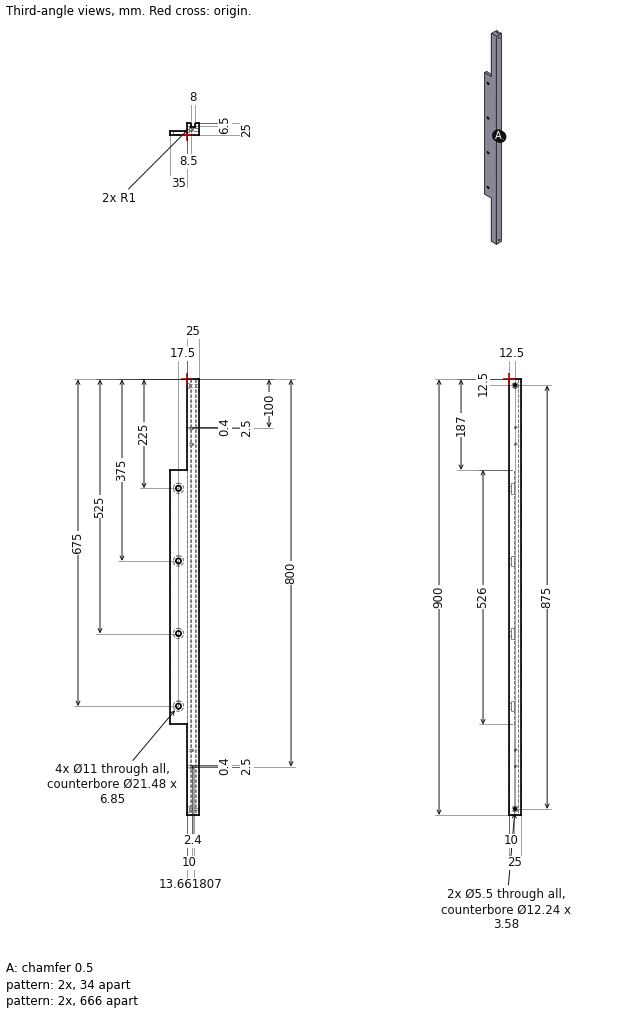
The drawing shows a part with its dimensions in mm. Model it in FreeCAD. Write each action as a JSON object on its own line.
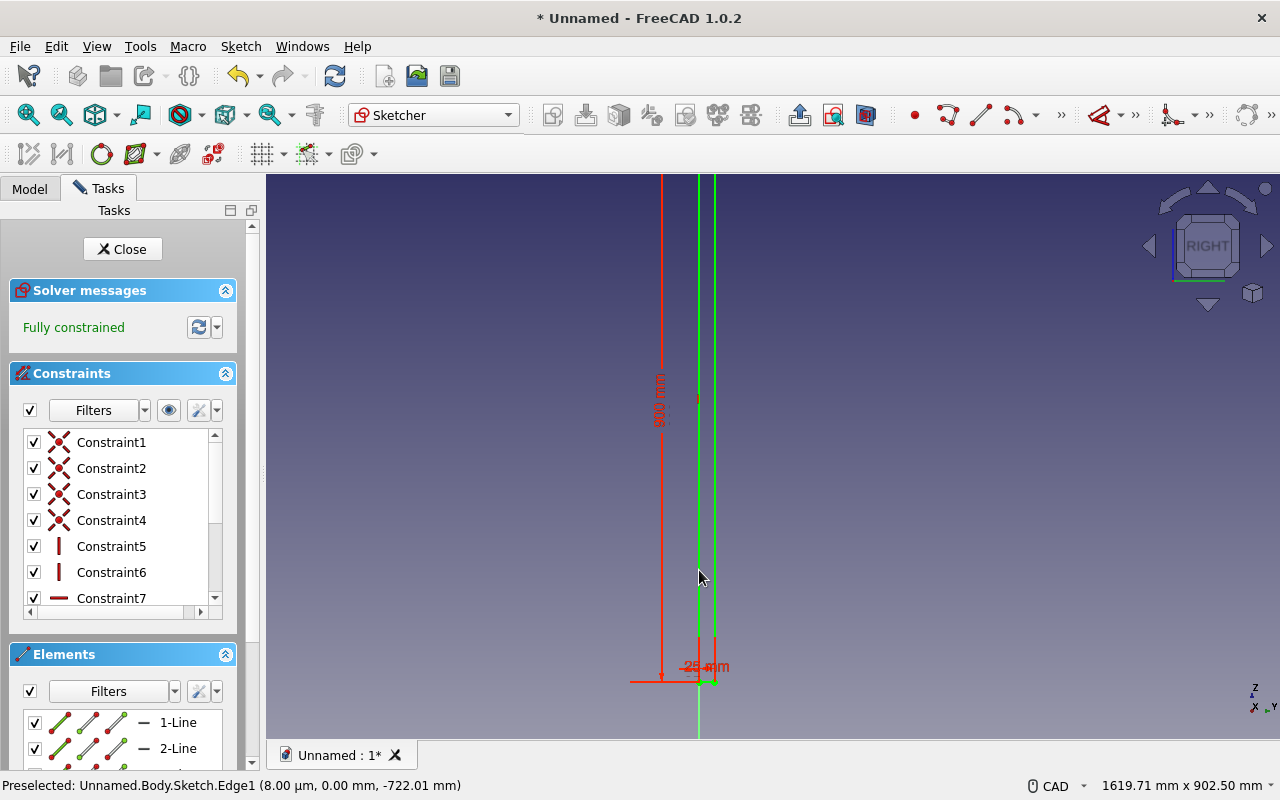
{"action": "left_click", "coordinate": [123, 249]}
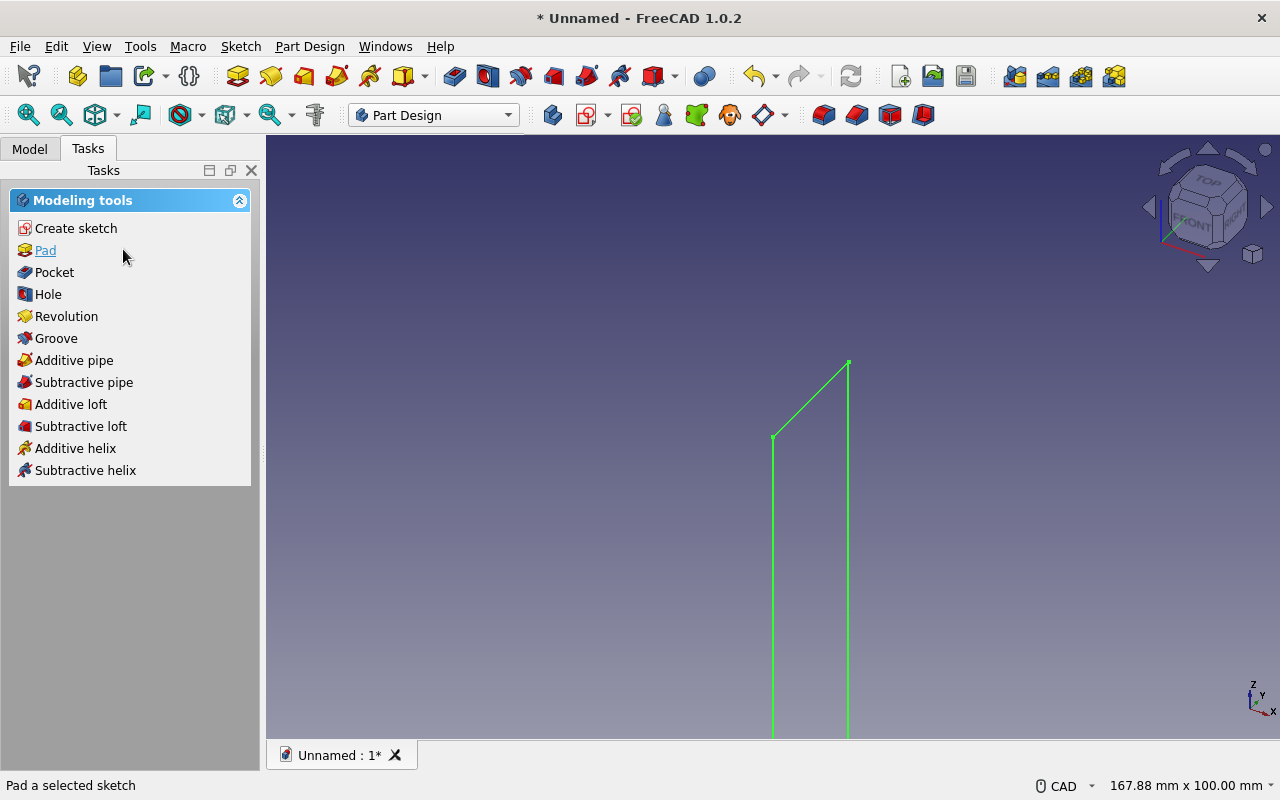
{"action": "left_click", "coordinate": [238, 76]}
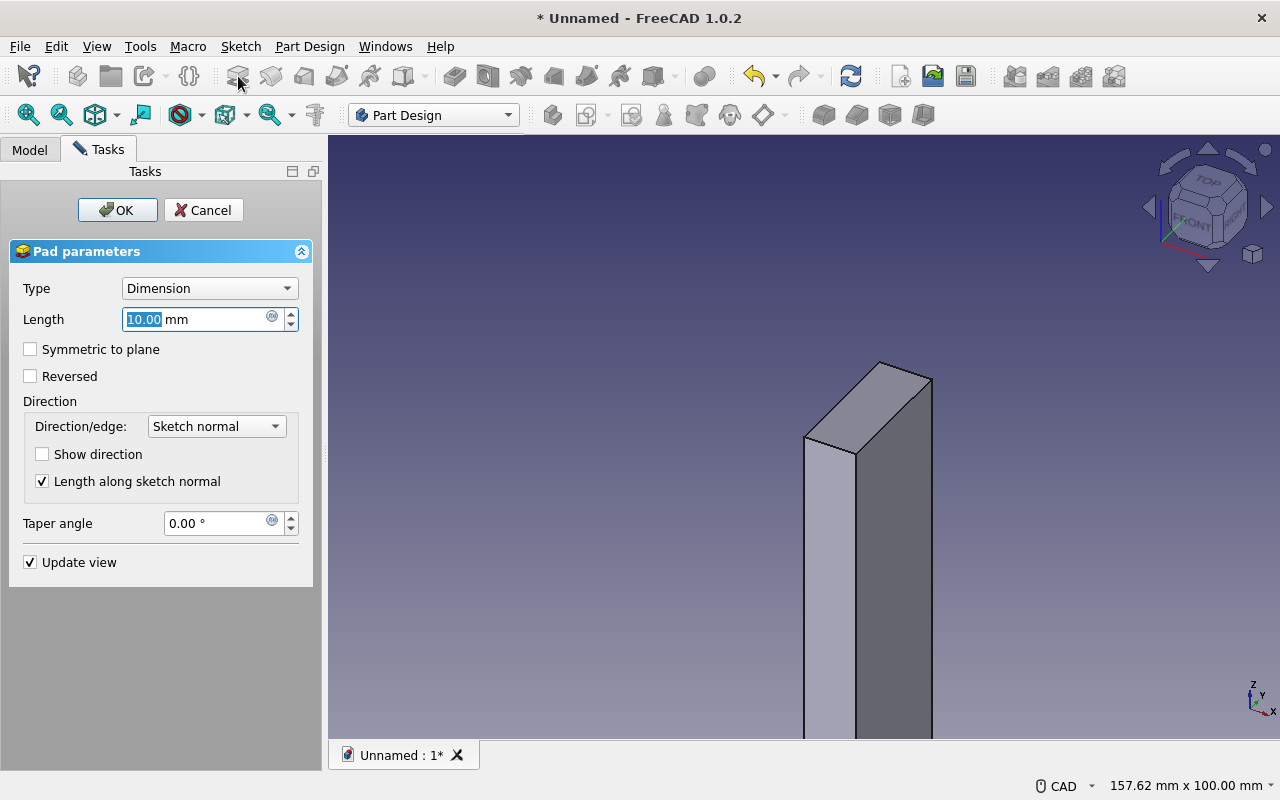
{"action": "type", "text": "25"}
{"action": "key", "text": "Tab"}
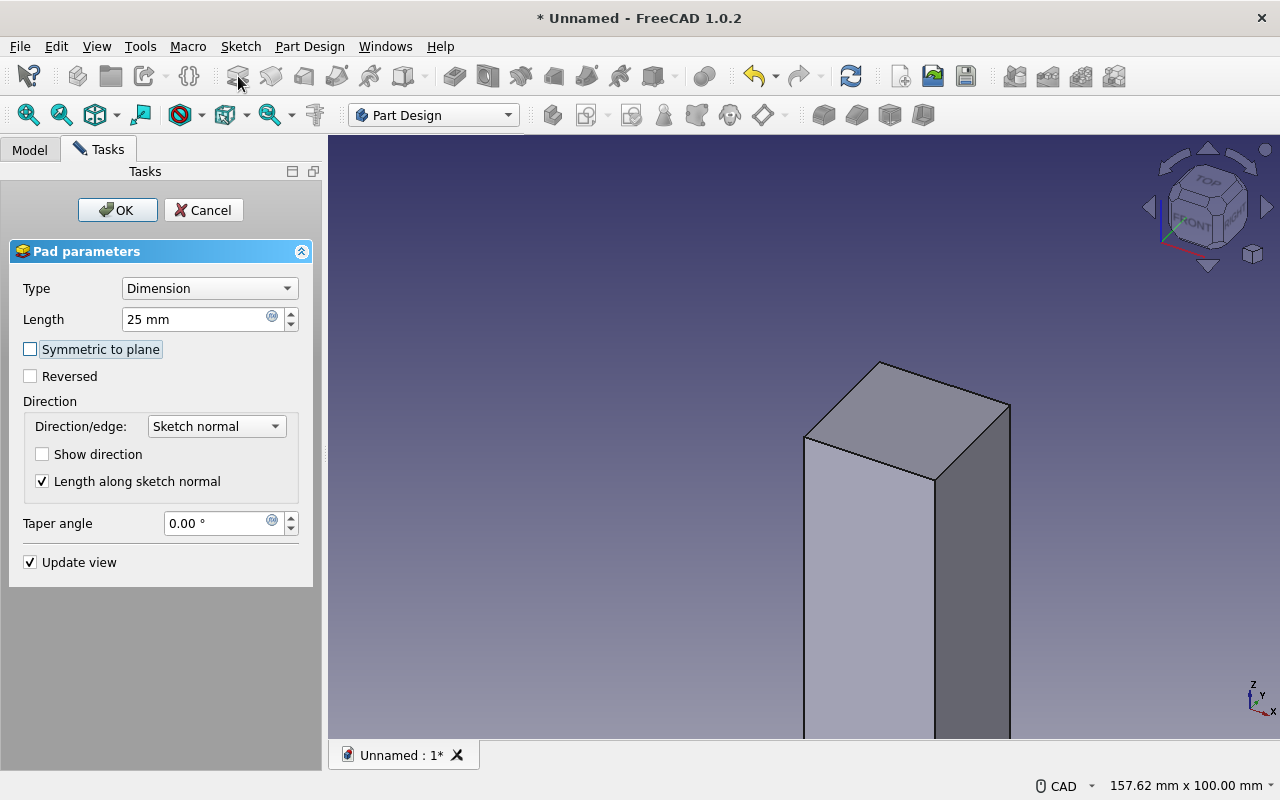
{"action": "left_click", "coordinate": [118, 210]}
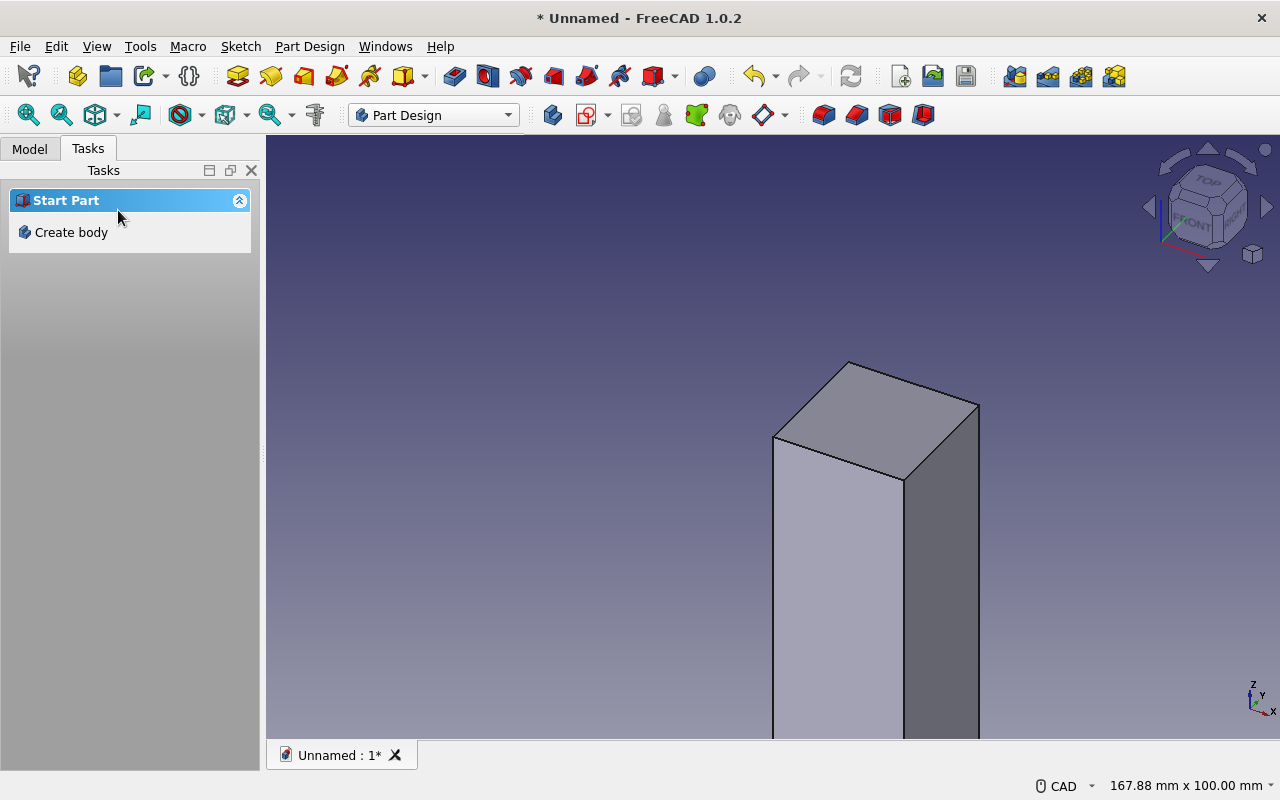
{"action": "key", "text": "v f"}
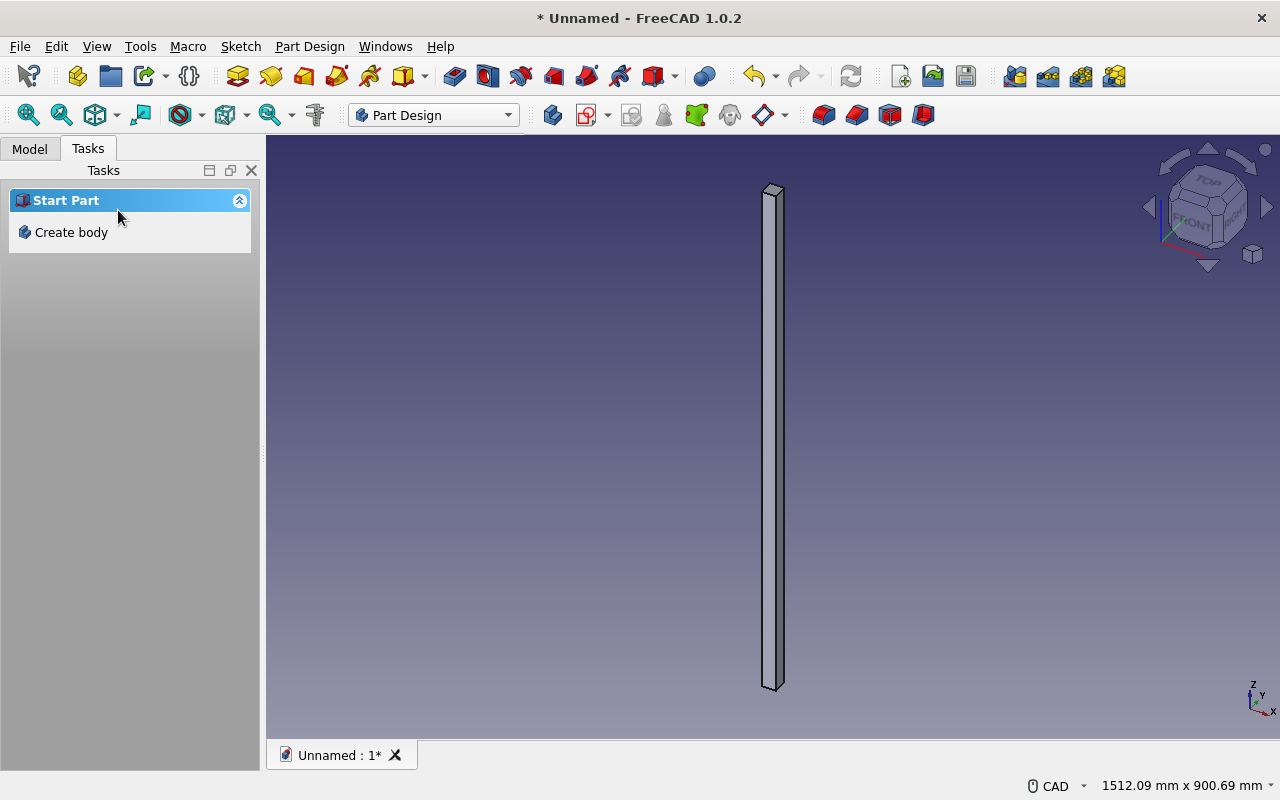
{"action": "left_click", "coordinate": [586, 116]}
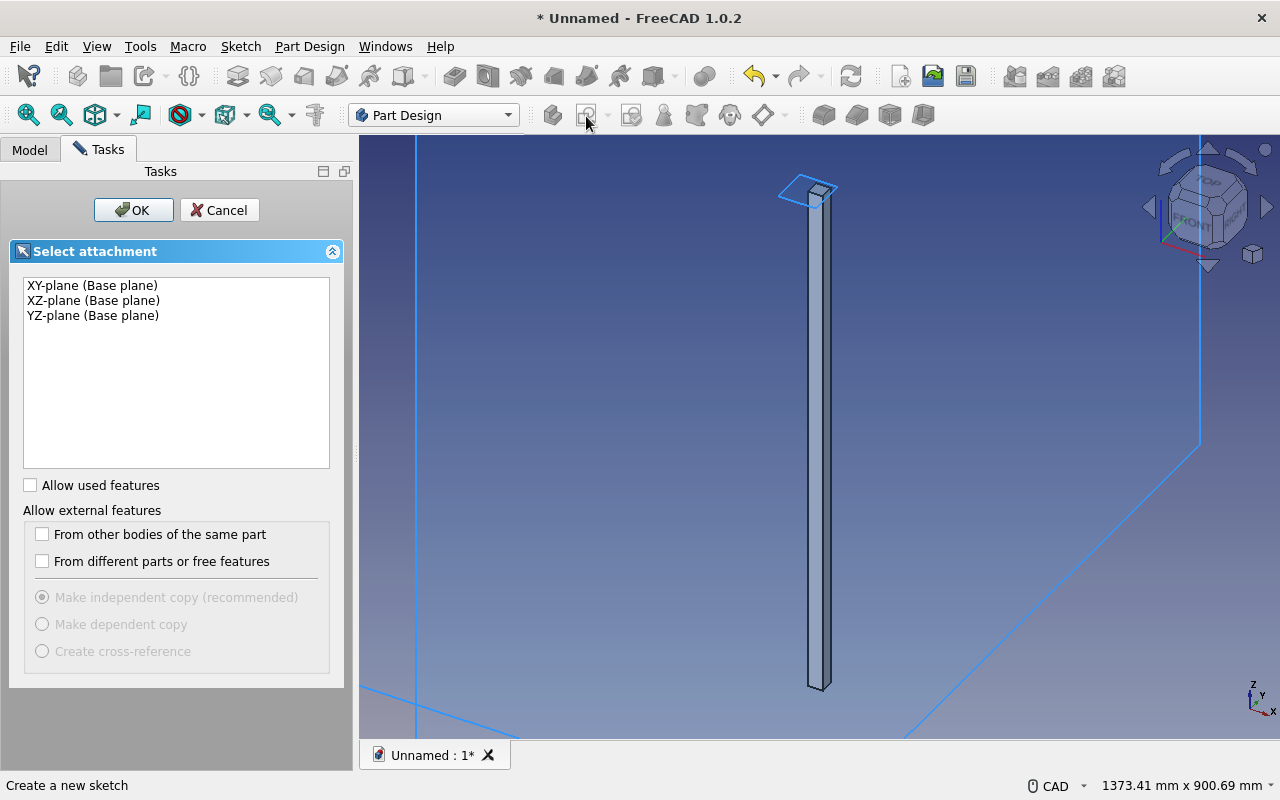
{"action": "left_click", "coordinate": [84, 316]}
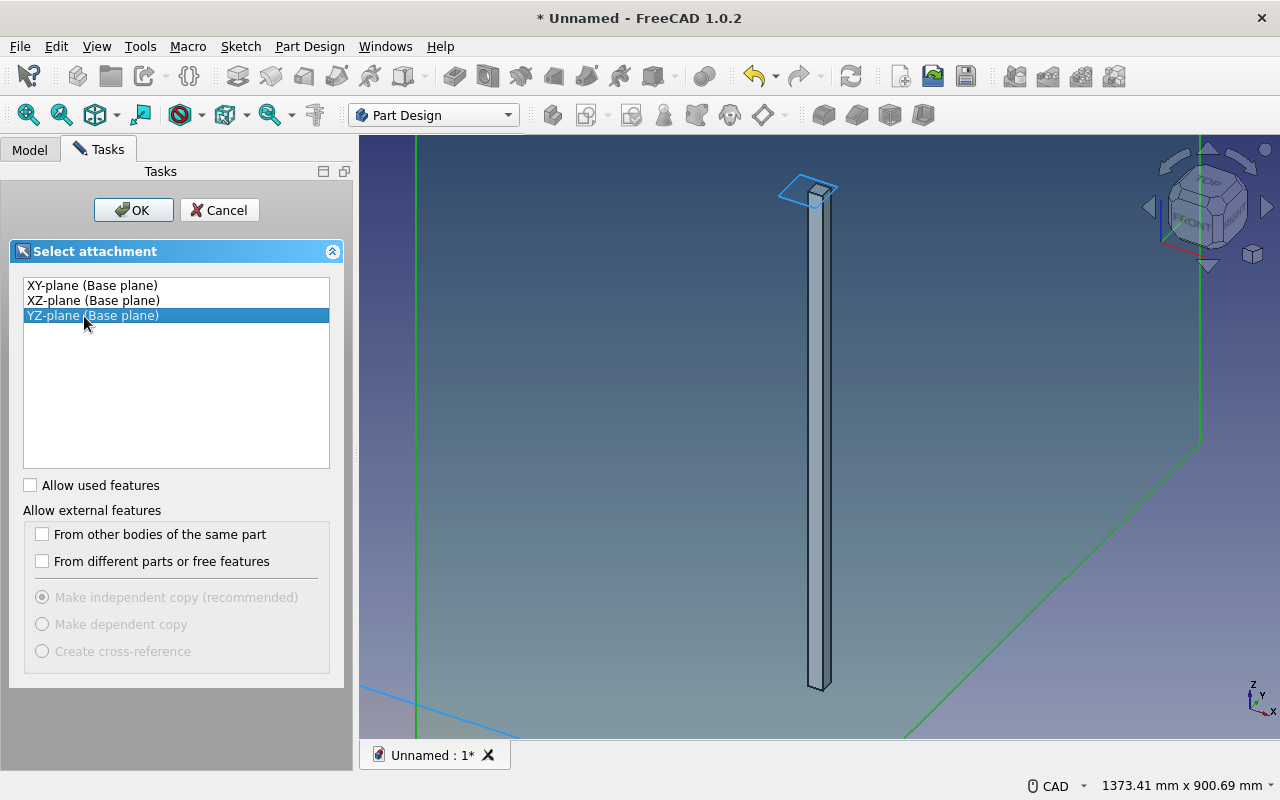
{"action": "left_click", "coordinate": [134, 210]}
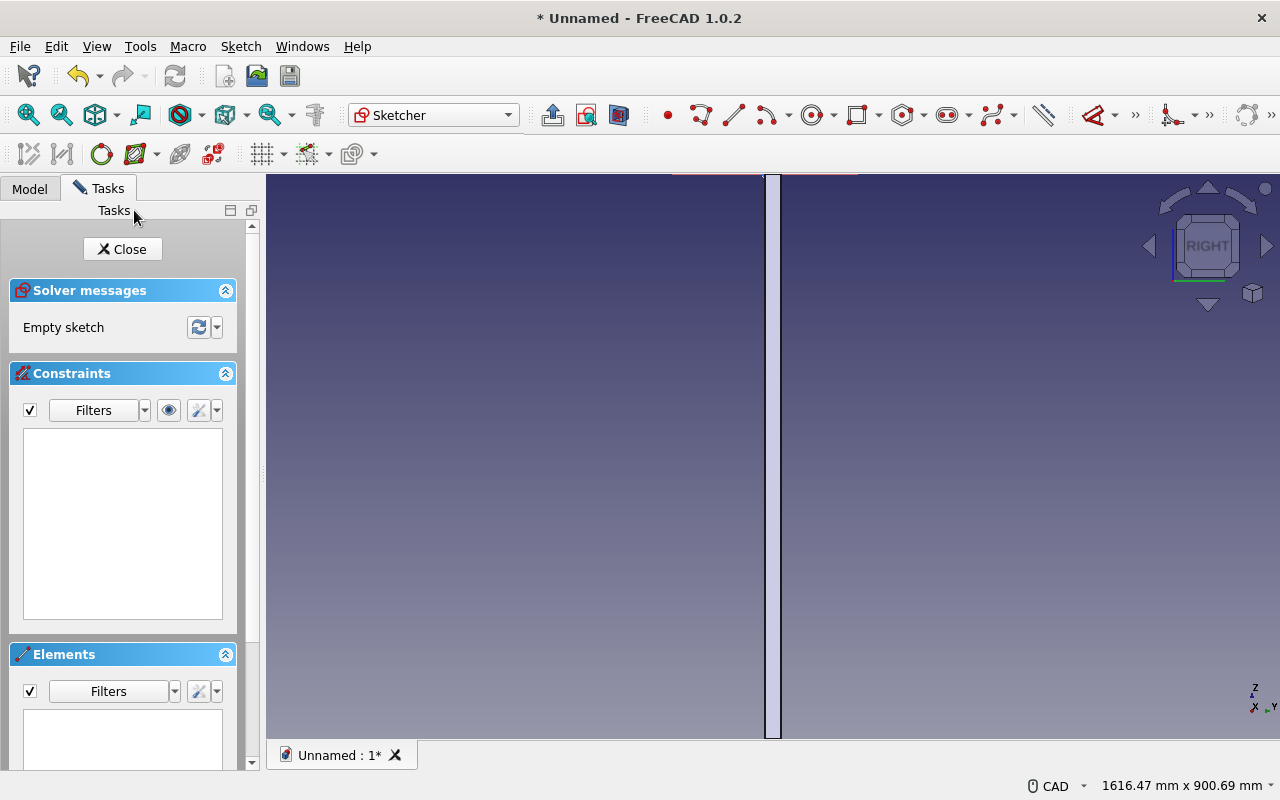
{"action": "left_click", "coordinate": [619, 116]}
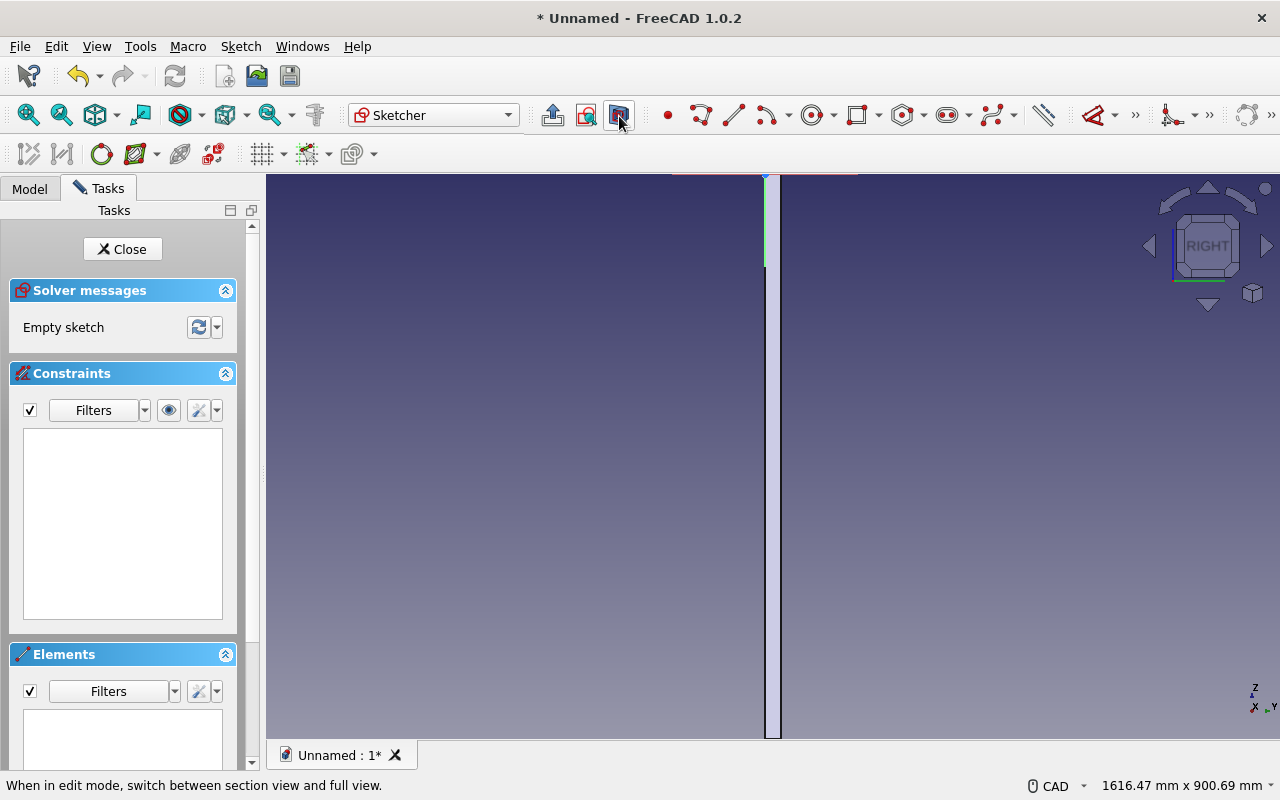
{"action": "scroll", "coordinate": [416, 711], "scroll_direction": "down", "scroll_amount": 1}